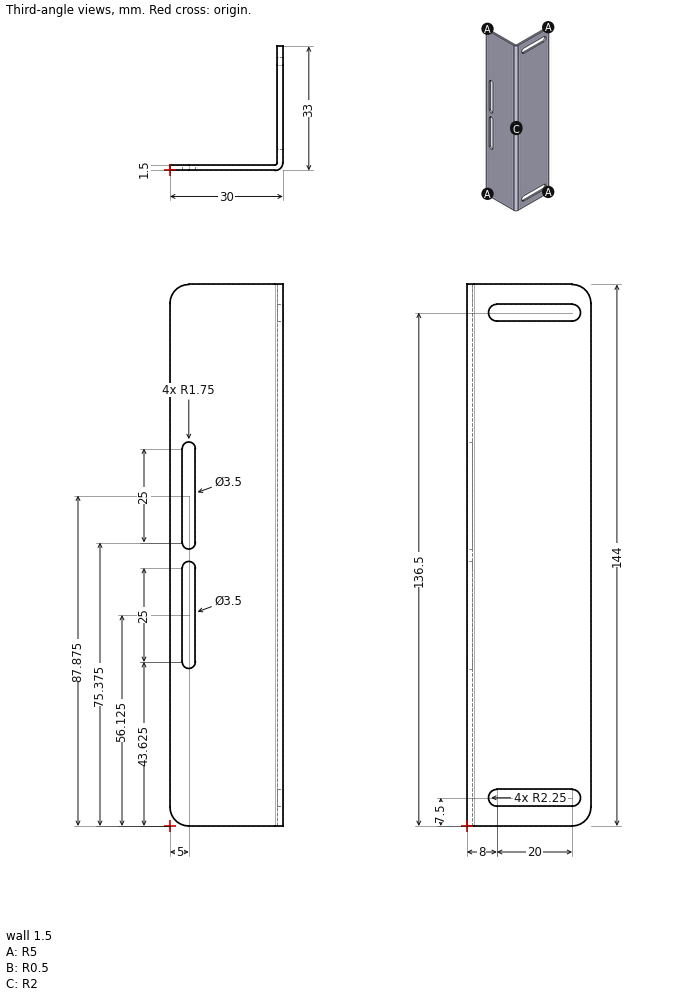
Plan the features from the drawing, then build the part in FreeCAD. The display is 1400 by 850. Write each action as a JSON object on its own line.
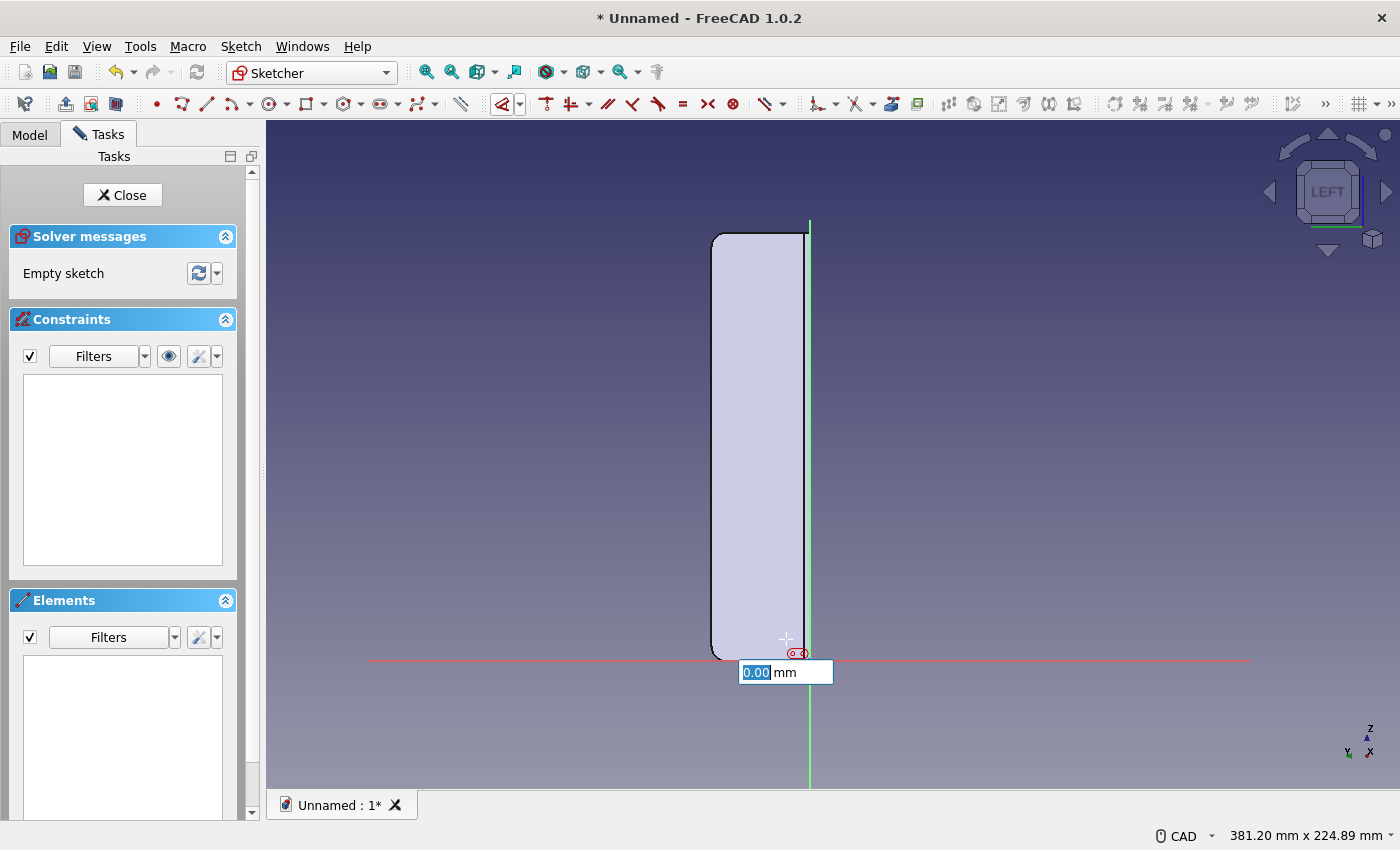
{"action": "scroll", "coordinate": [756, 645], "scroll_direction": "up", "scroll_amount": 5}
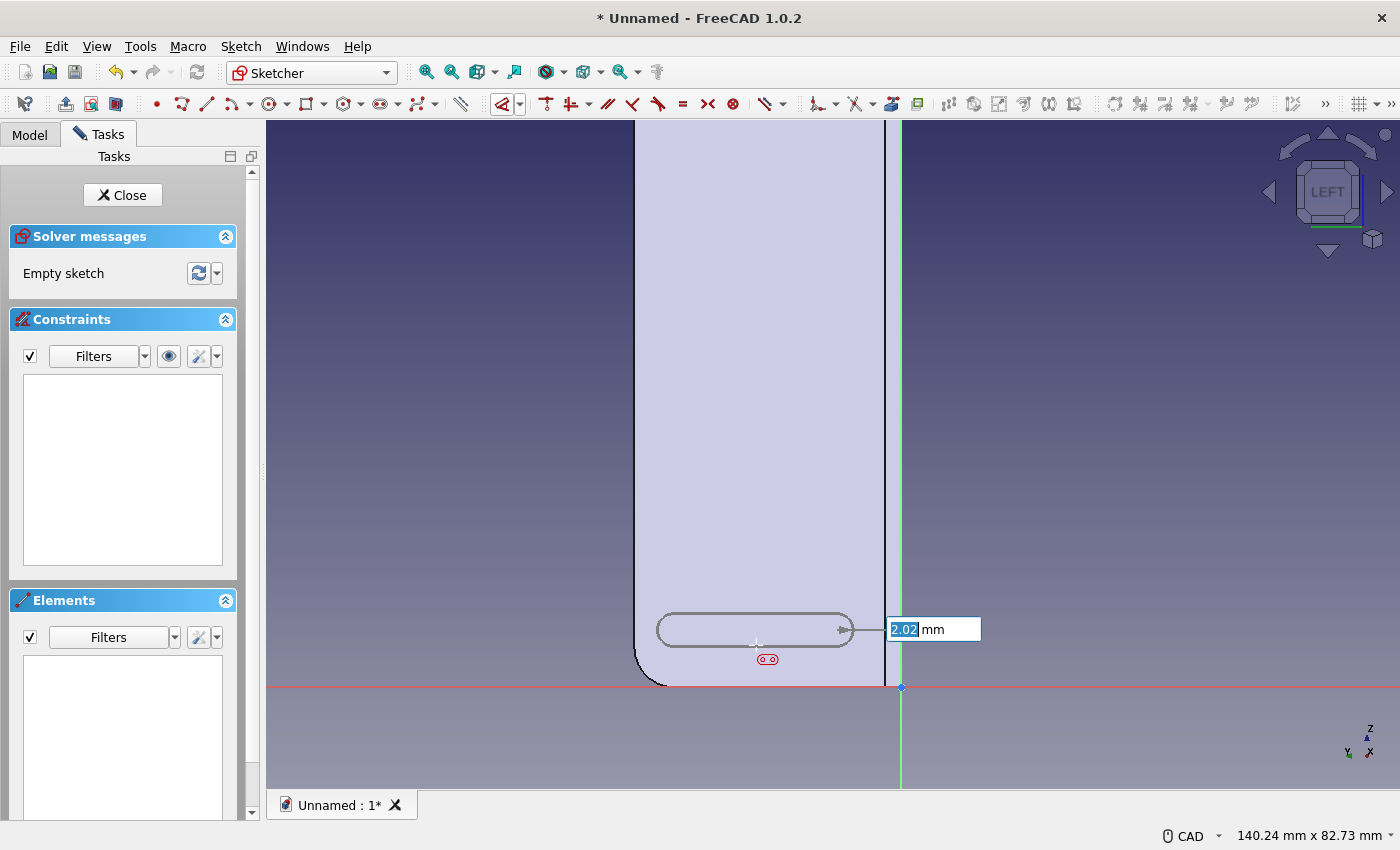
{"action": "left_click", "coordinate": [756, 645]}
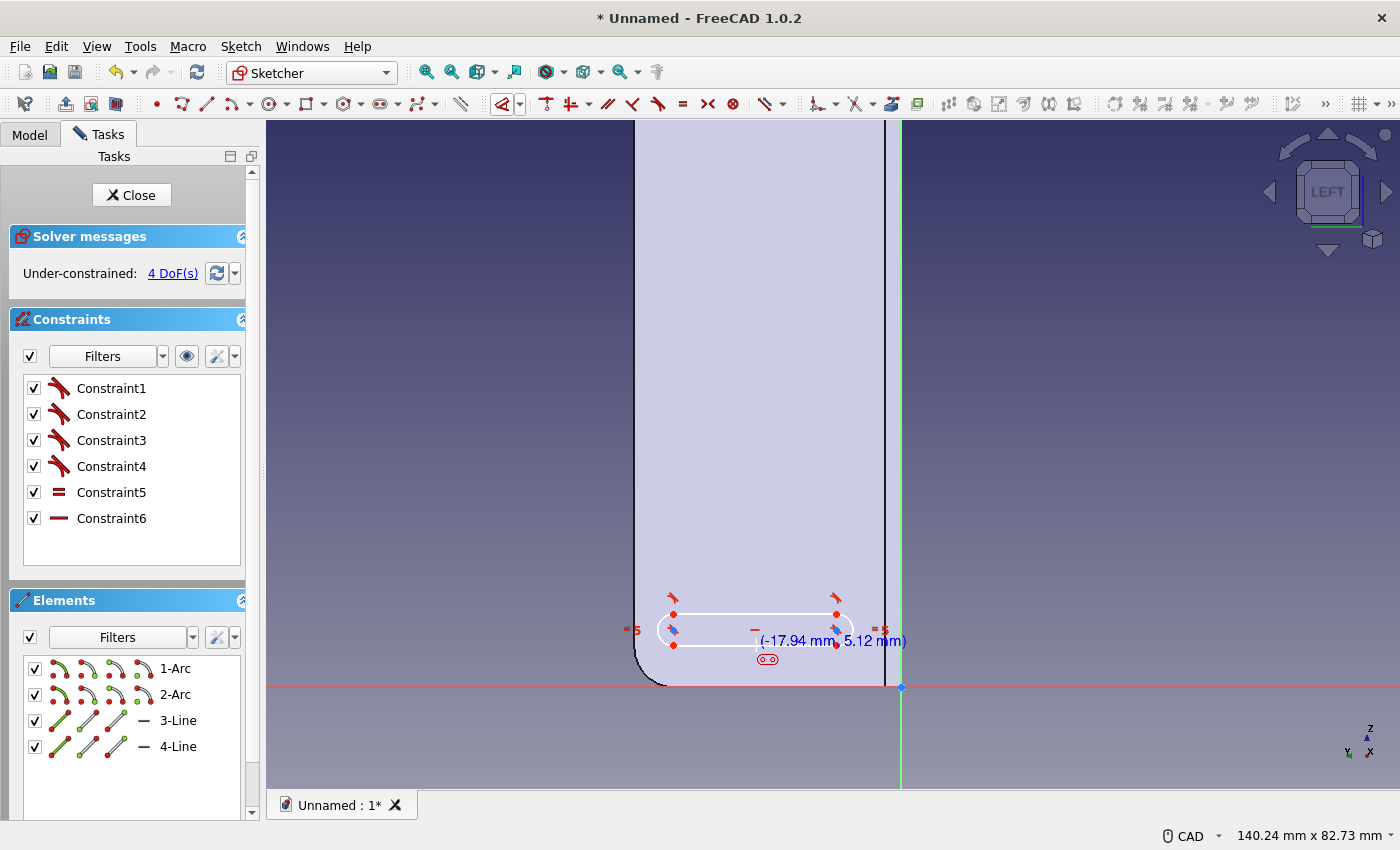
{"action": "scroll", "coordinate": [756, 645], "scroll_direction": "down", "scroll_amount": 5}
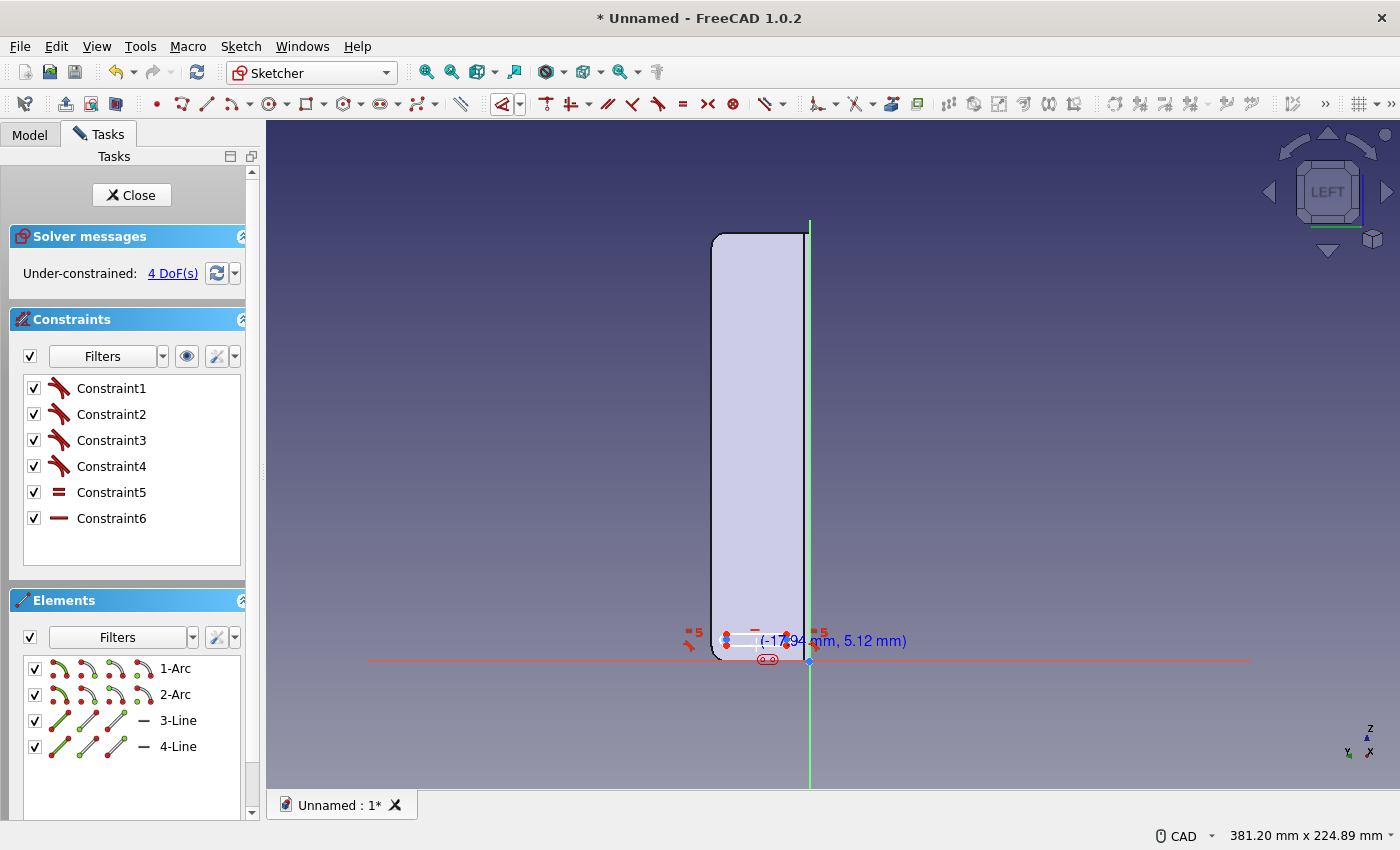
{"action": "scroll", "coordinate": [726, 255], "scroll_direction": "up", "scroll_amount": 7}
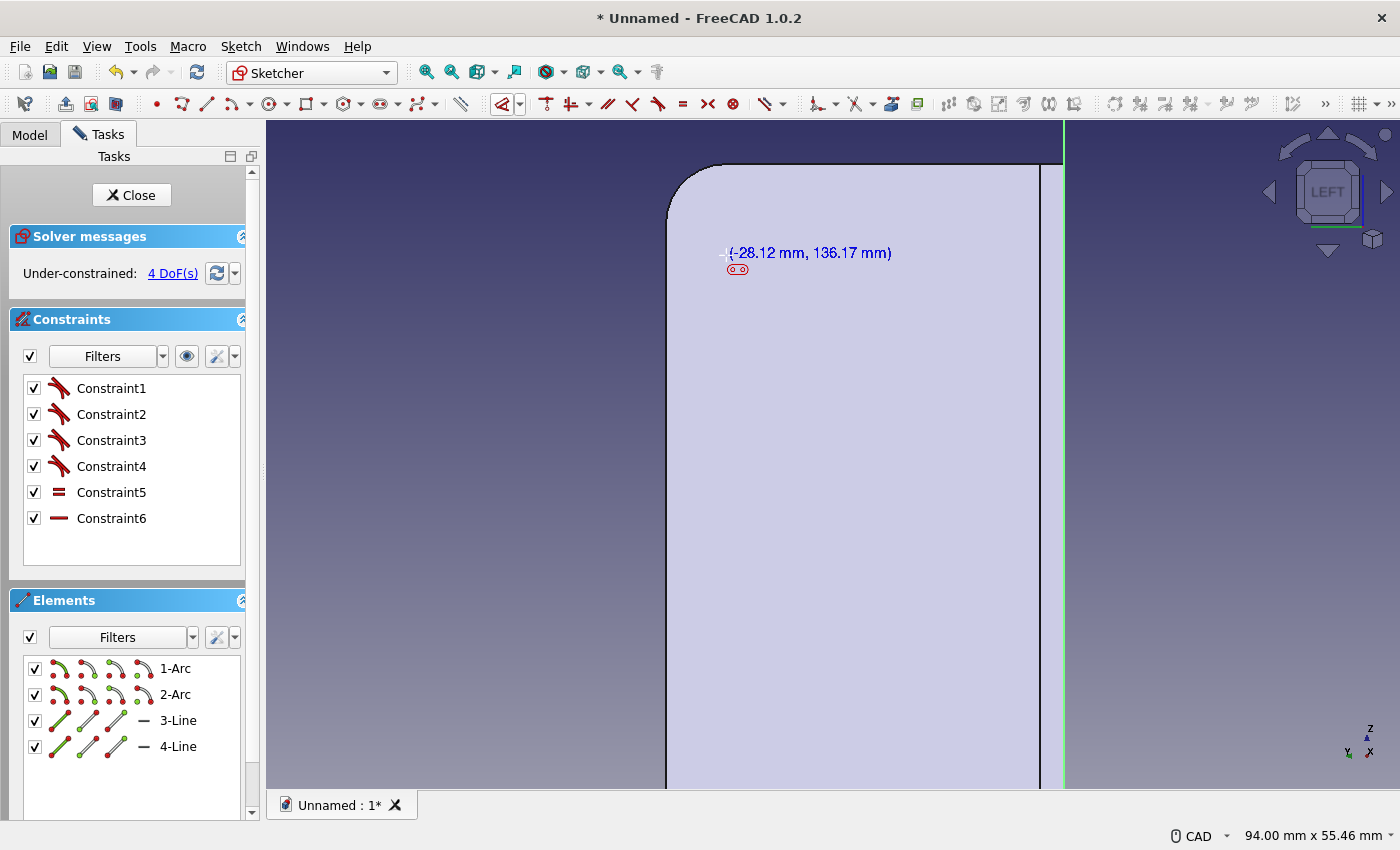
{"action": "scroll", "coordinate": [726, 255], "scroll_direction": "down", "scroll_amount": 7}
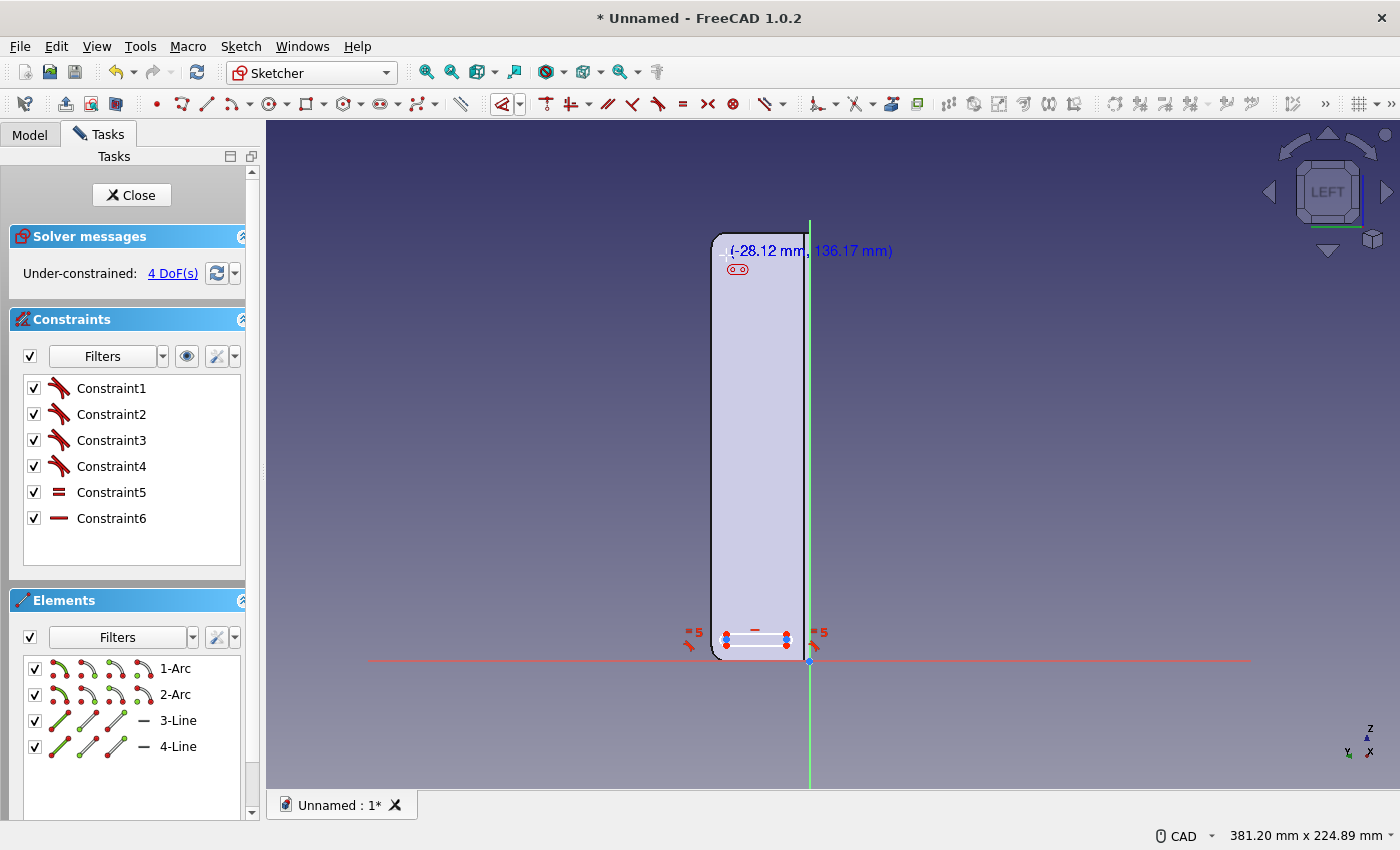
{"action": "left_click", "coordinate": [726, 255]}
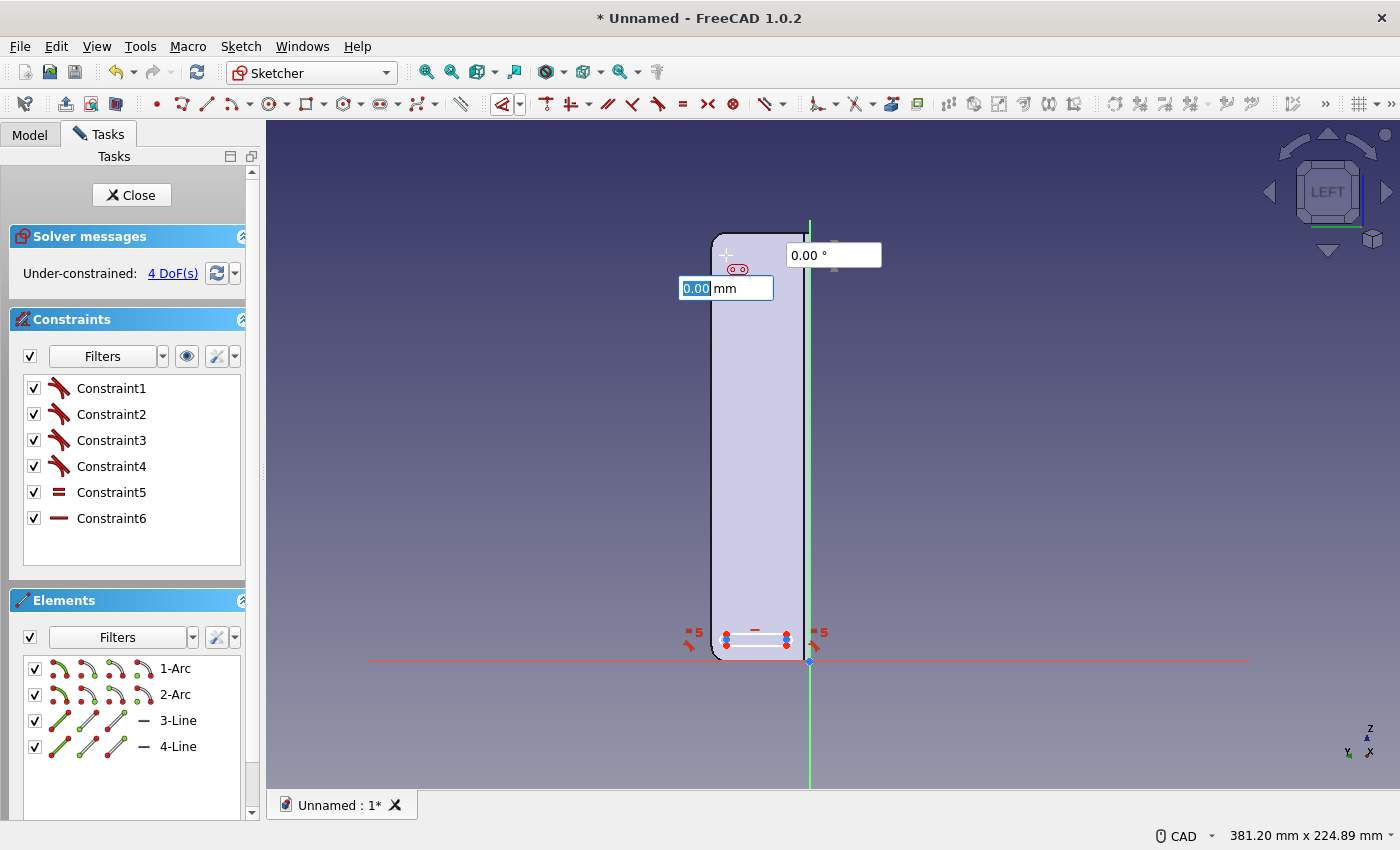
{"action": "left_click", "coordinate": [786, 255]}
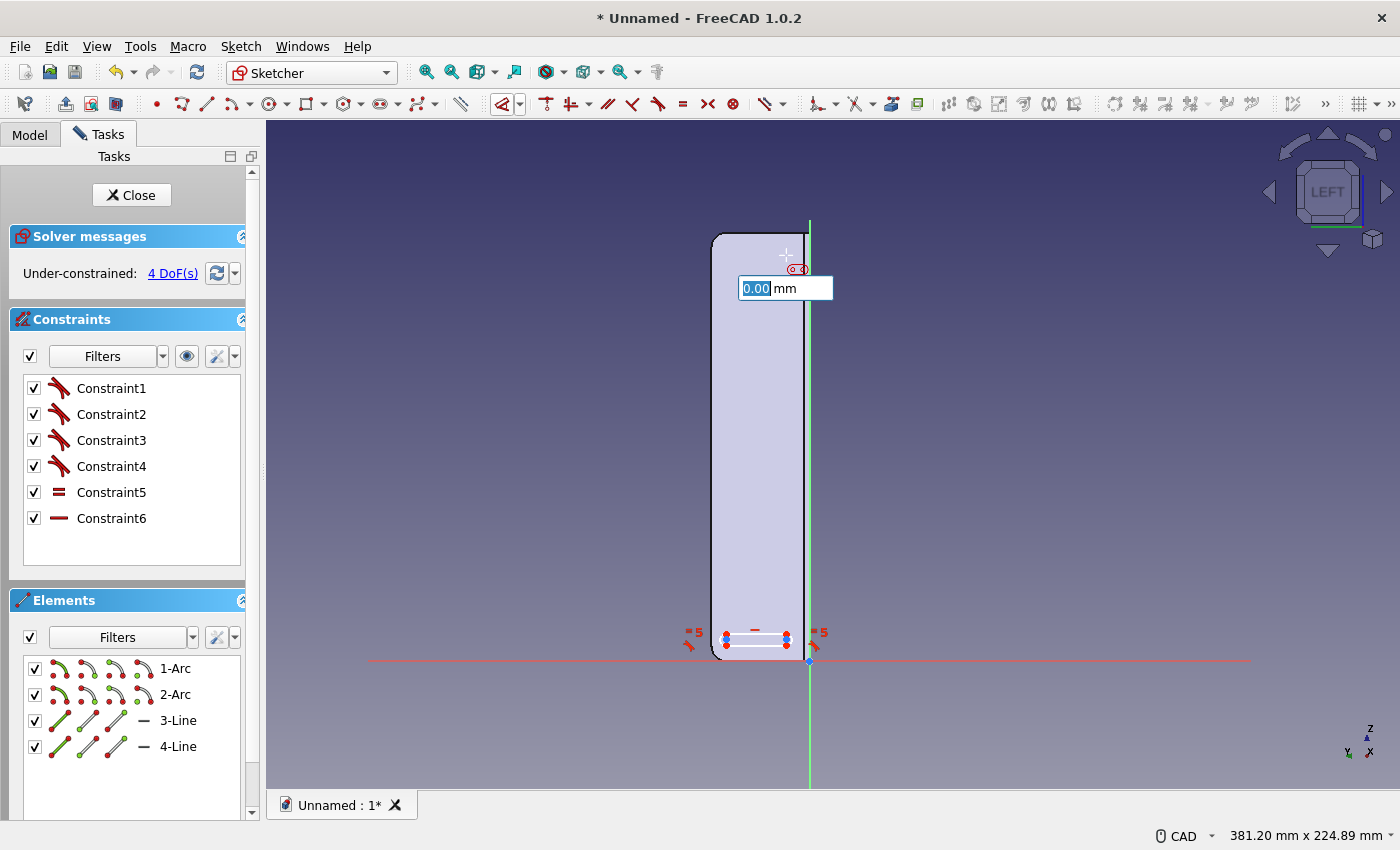
{"action": "scroll", "coordinate": [756, 248], "scroll_direction": "up", "scroll_amount": 5}